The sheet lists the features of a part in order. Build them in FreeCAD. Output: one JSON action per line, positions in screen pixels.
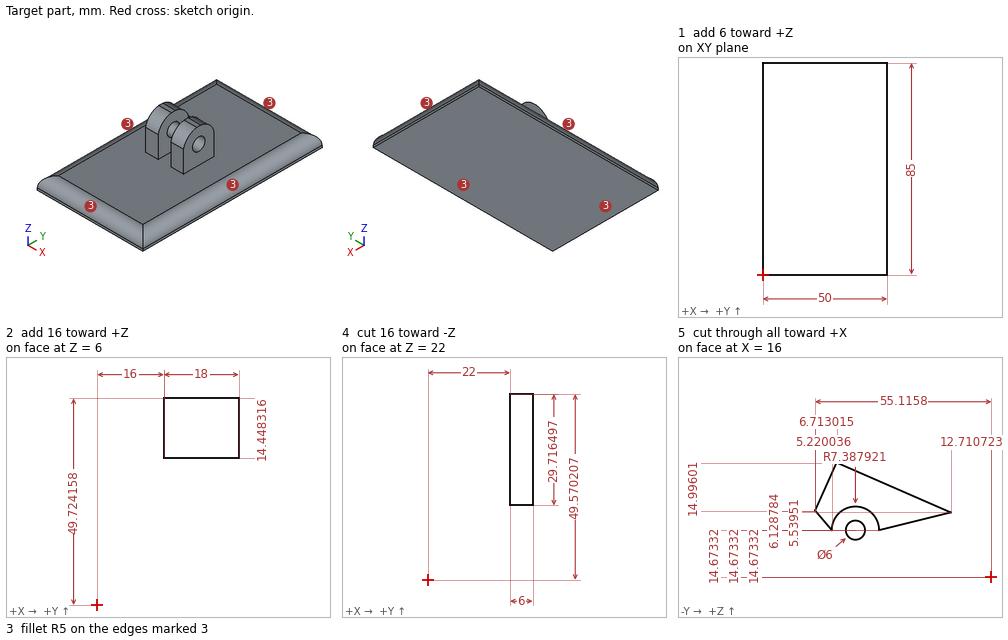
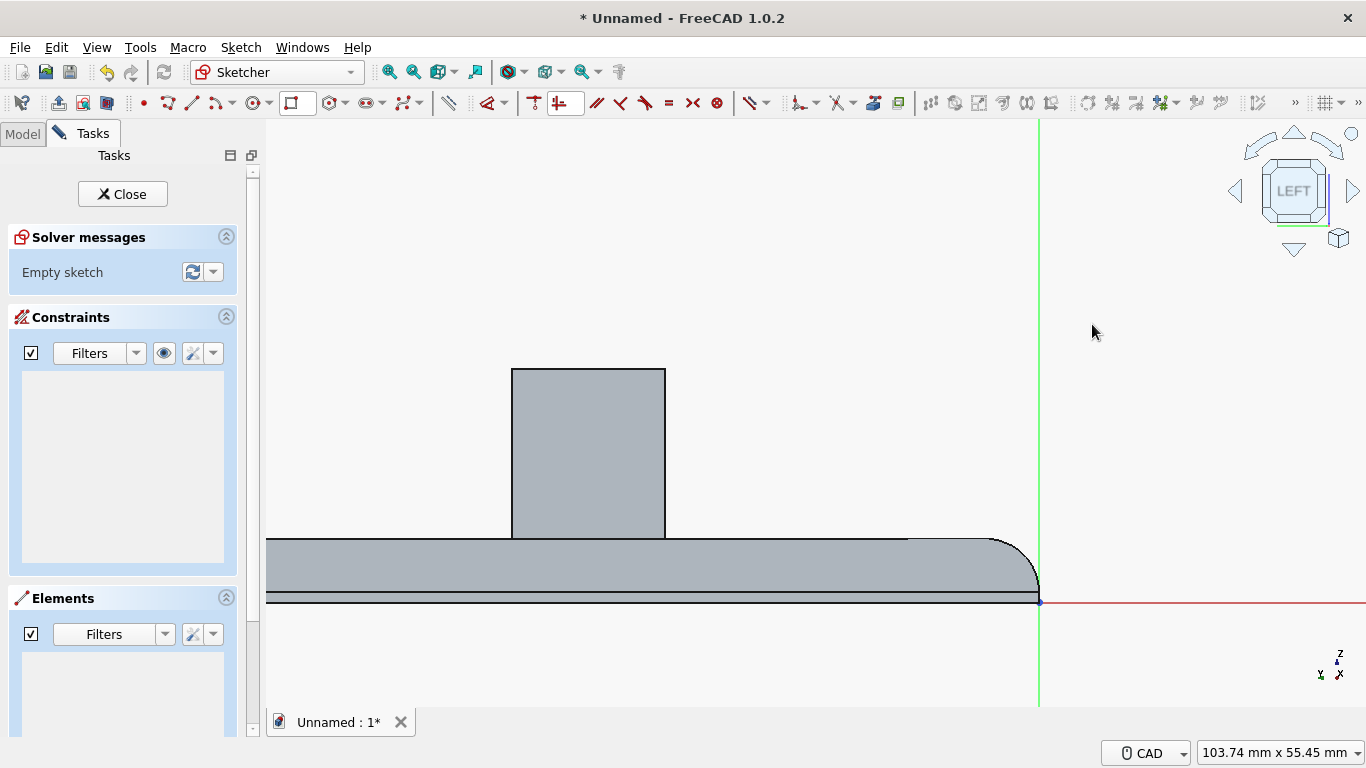
{"action": "left_click", "coordinate": [168, 104]}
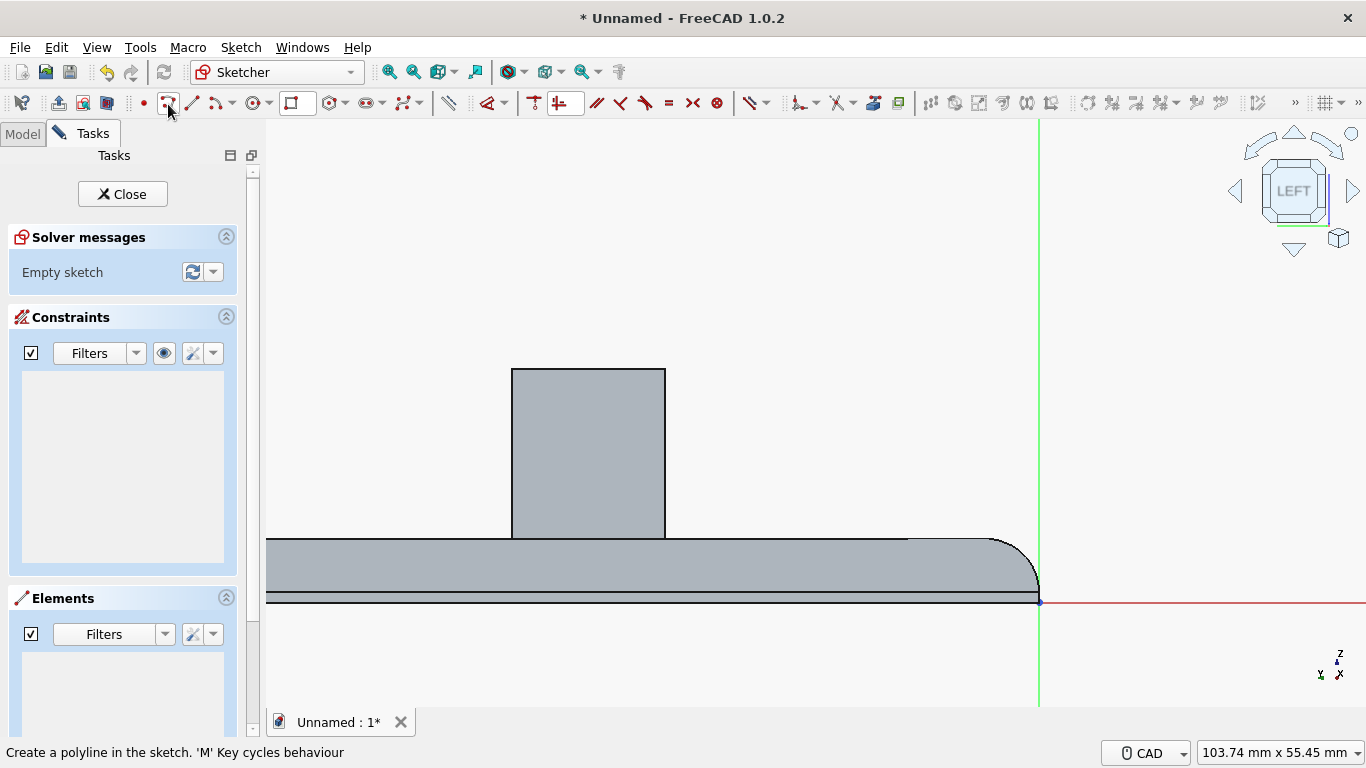
{"action": "left_click", "coordinate": [667, 447]}
{"action": "left_click", "coordinate": [904, 388]}
{"action": "left_click", "coordinate": [526, 223]}
{"action": "left_click", "coordinate": [455, 382]}
{"action": "left_click", "coordinate": [510, 447]}
{"action": "right_click", "coordinate": [510, 447]}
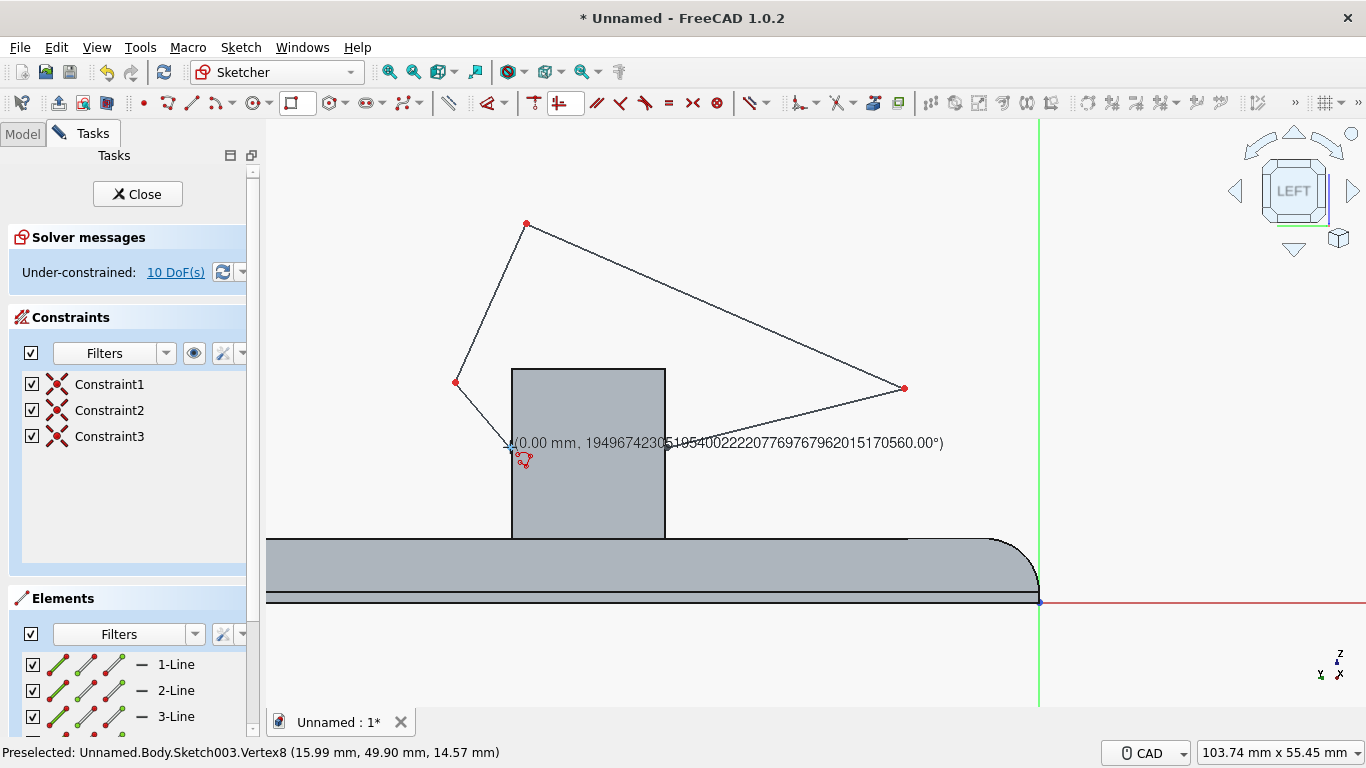
{"action": "key", "text": "g 3 a"}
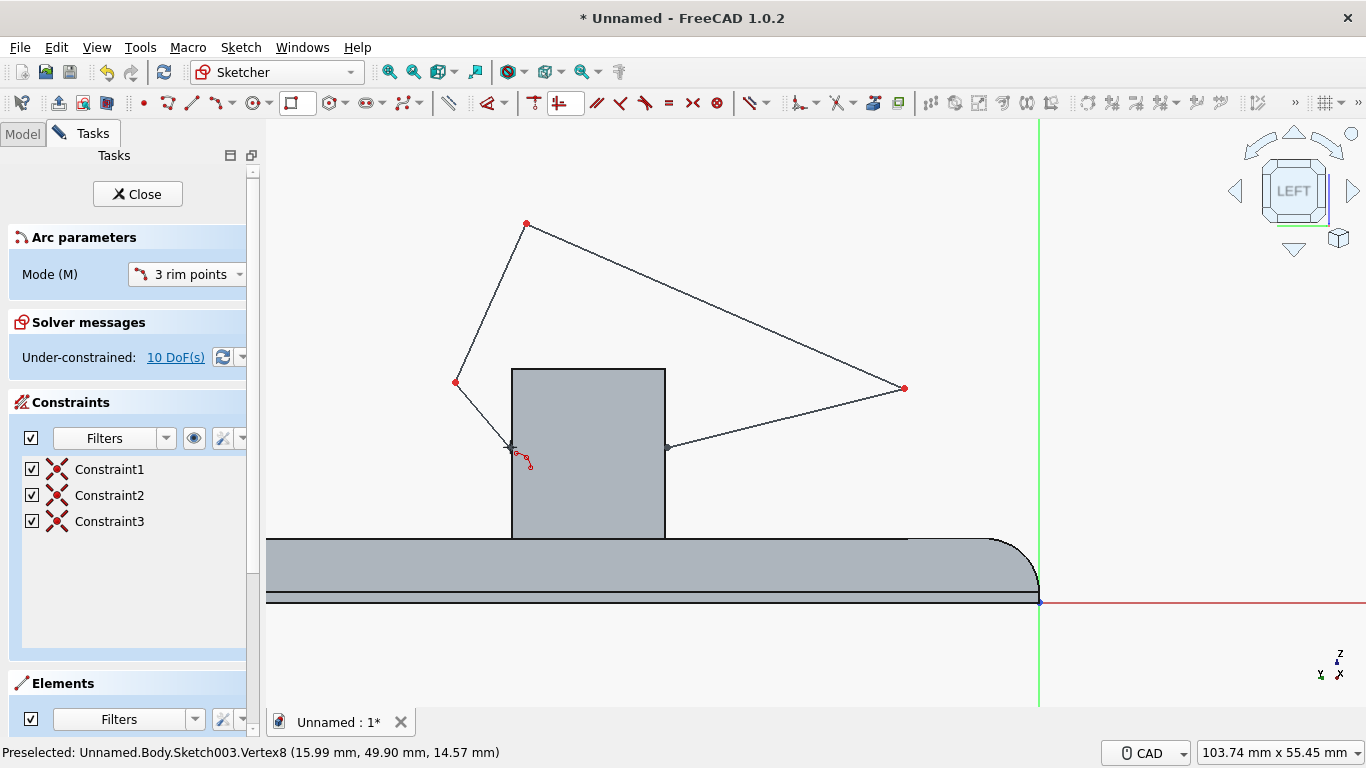
{"action": "left_click", "coordinate": [510, 448]}
{"action": "left_click", "coordinate": [667, 448]}
{"action": "left_click", "coordinate": [588, 369]}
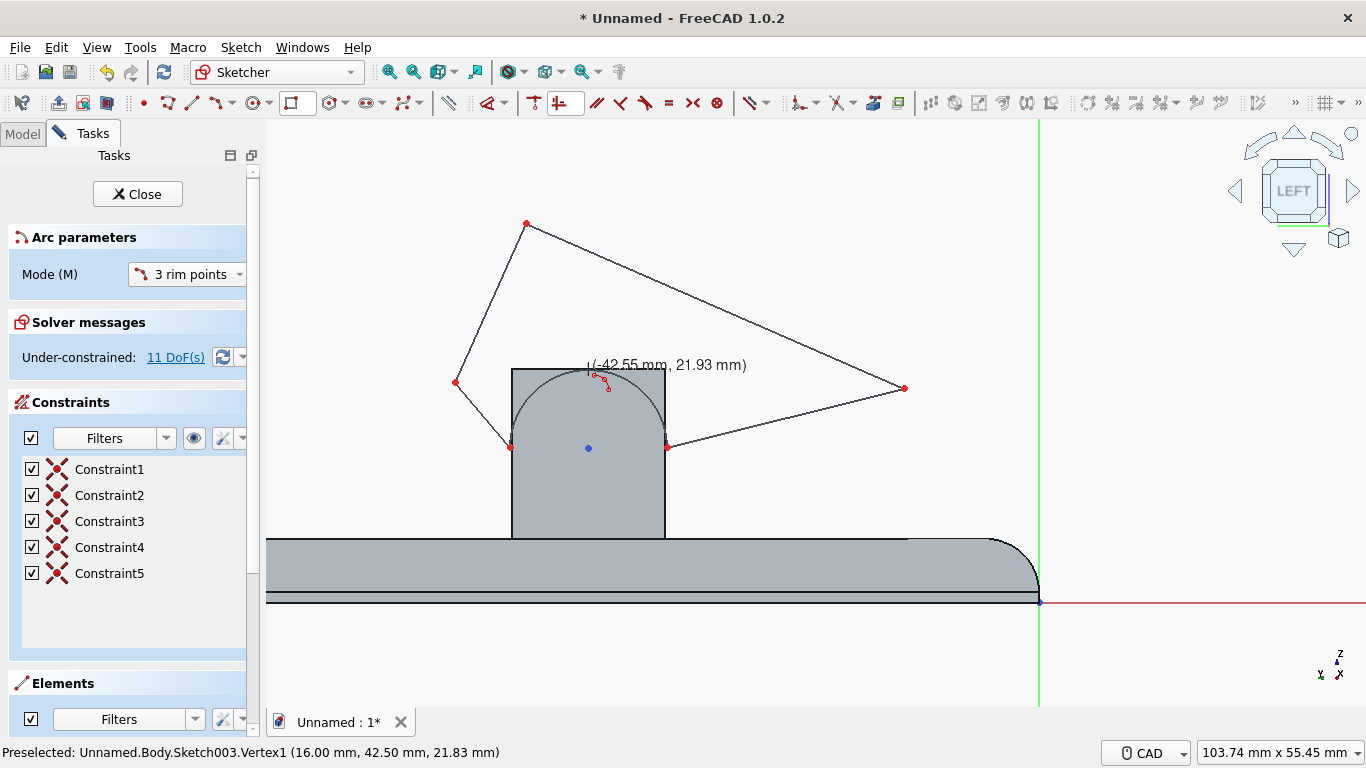
{"action": "left_click", "coordinate": [254, 104]}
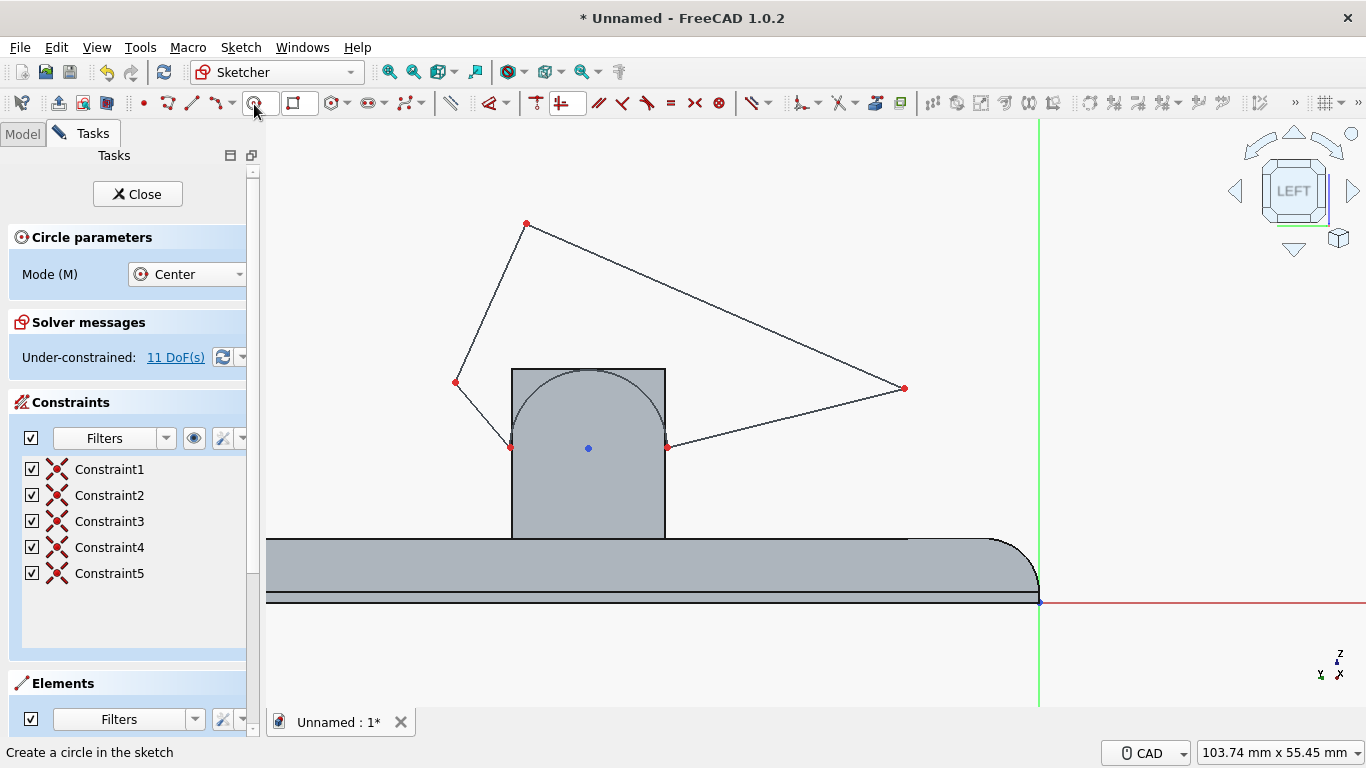
{"action": "left_click", "coordinate": [588, 447]}
{"action": "mouse_move", "coordinate": [611, 424]}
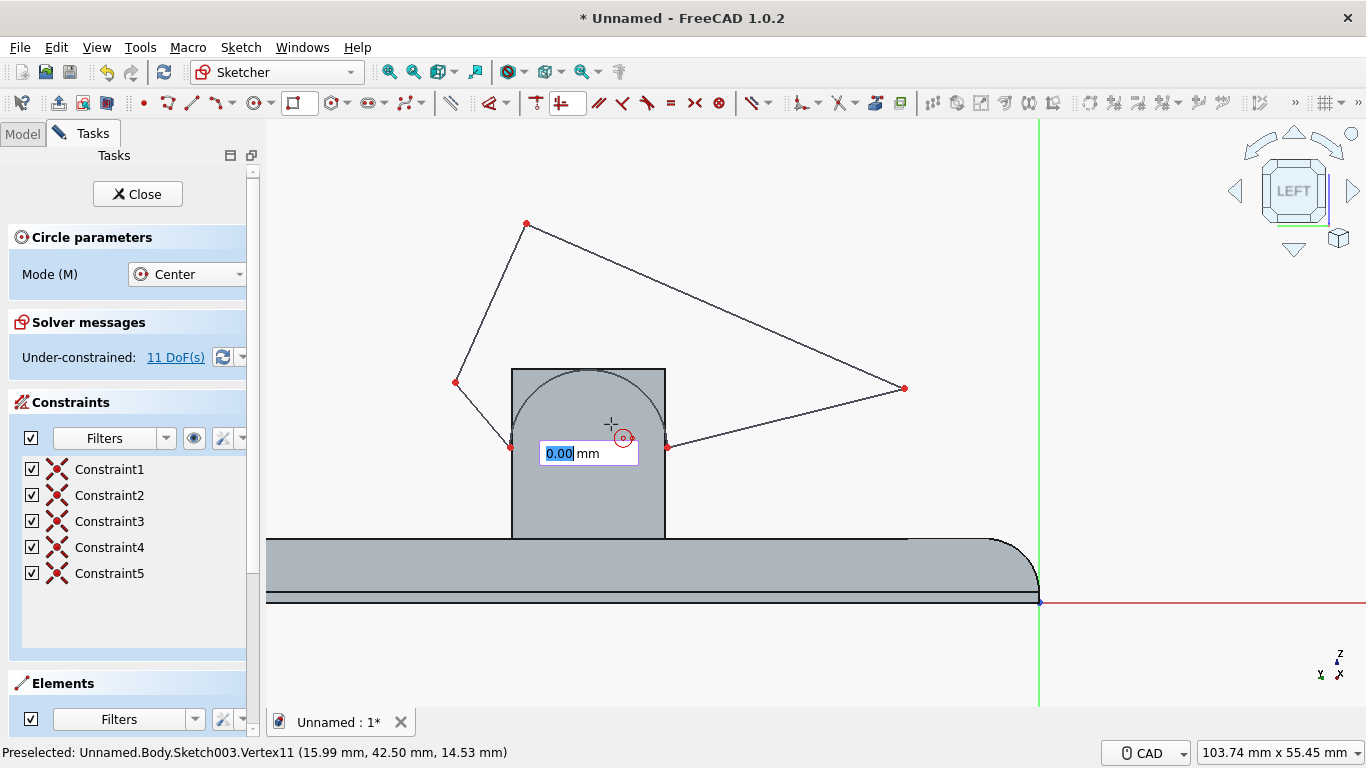
{"action": "type", "text": "6"}
{"action": "key", "text": "Return"}
{"action": "key", "text": "Escape"}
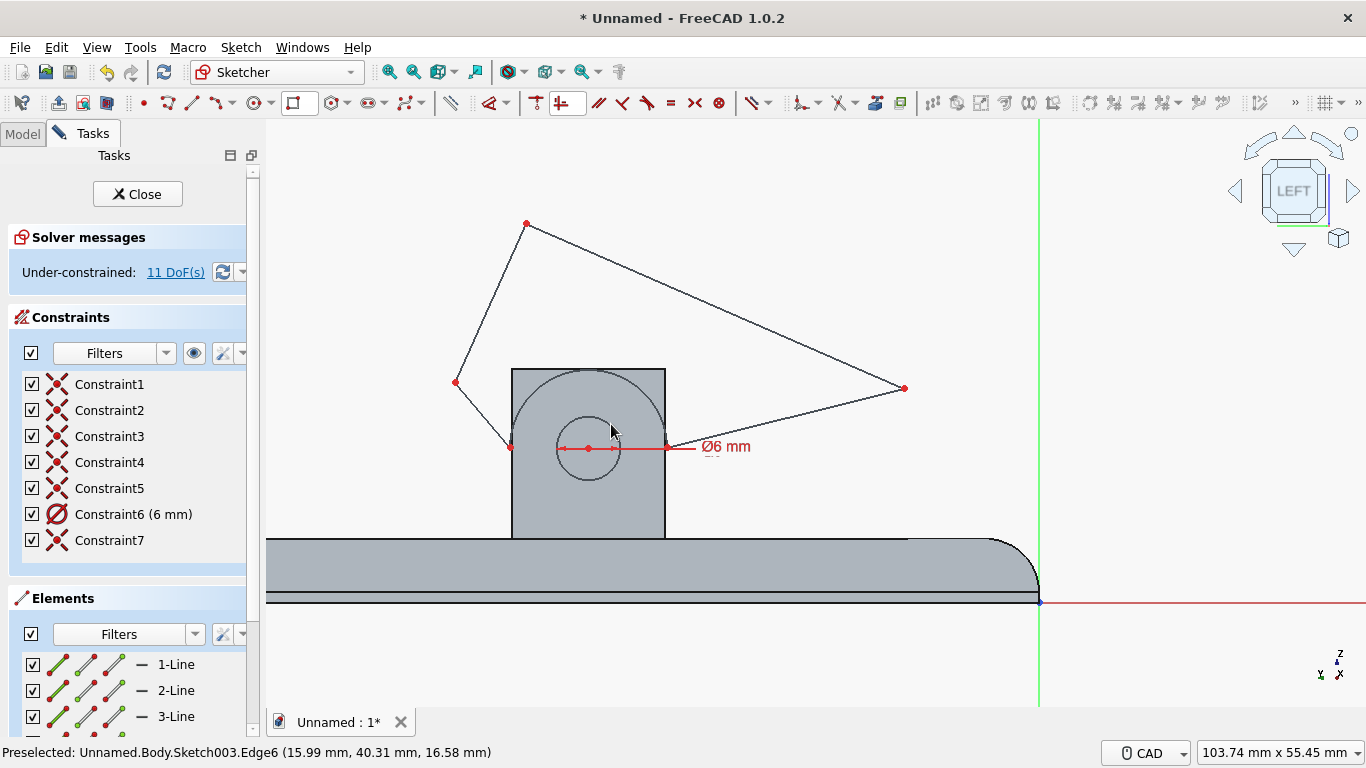
{"action": "left_click", "coordinate": [490, 104]}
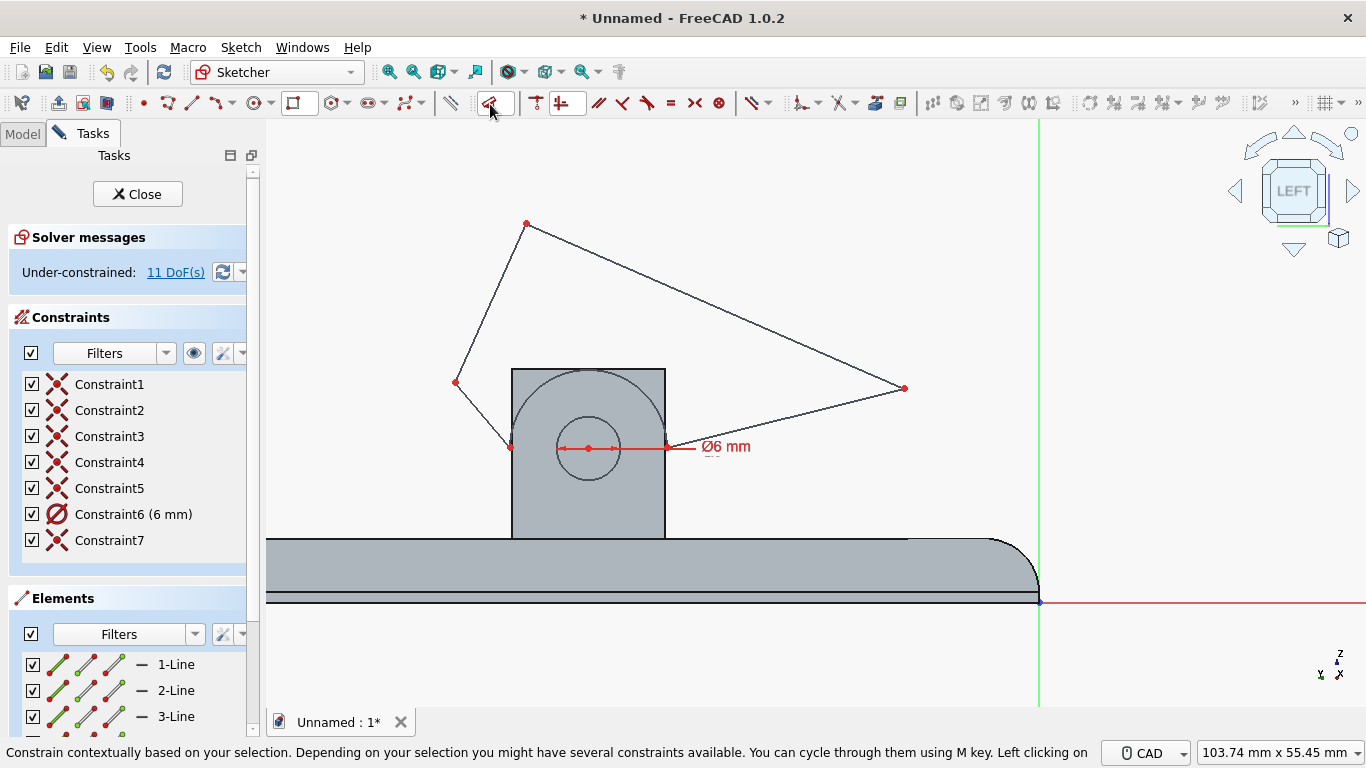
{"action": "left_click", "coordinate": [634, 385]}
{"action": "left_click", "coordinate": [653, 359]}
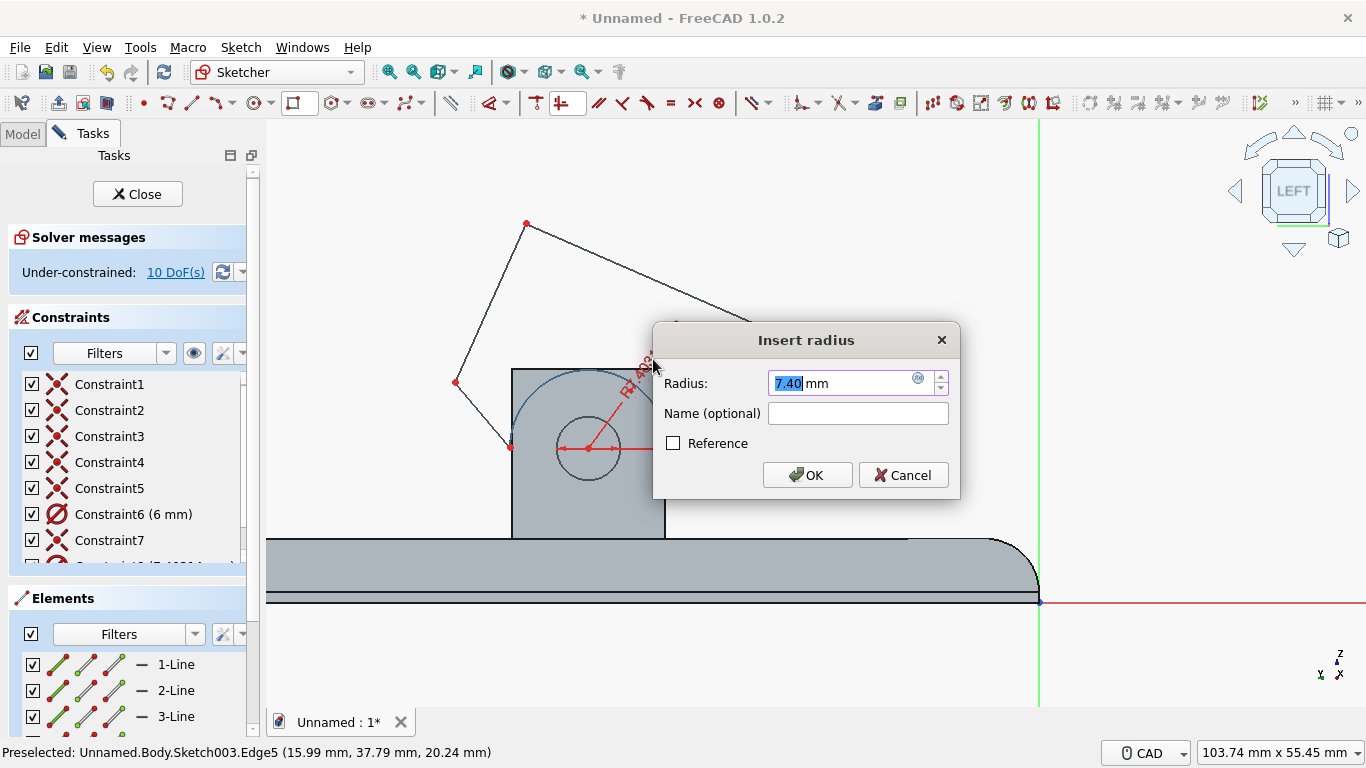
{"action": "type", "text": "7.387921"}
{"action": "key", "text": "Return"}